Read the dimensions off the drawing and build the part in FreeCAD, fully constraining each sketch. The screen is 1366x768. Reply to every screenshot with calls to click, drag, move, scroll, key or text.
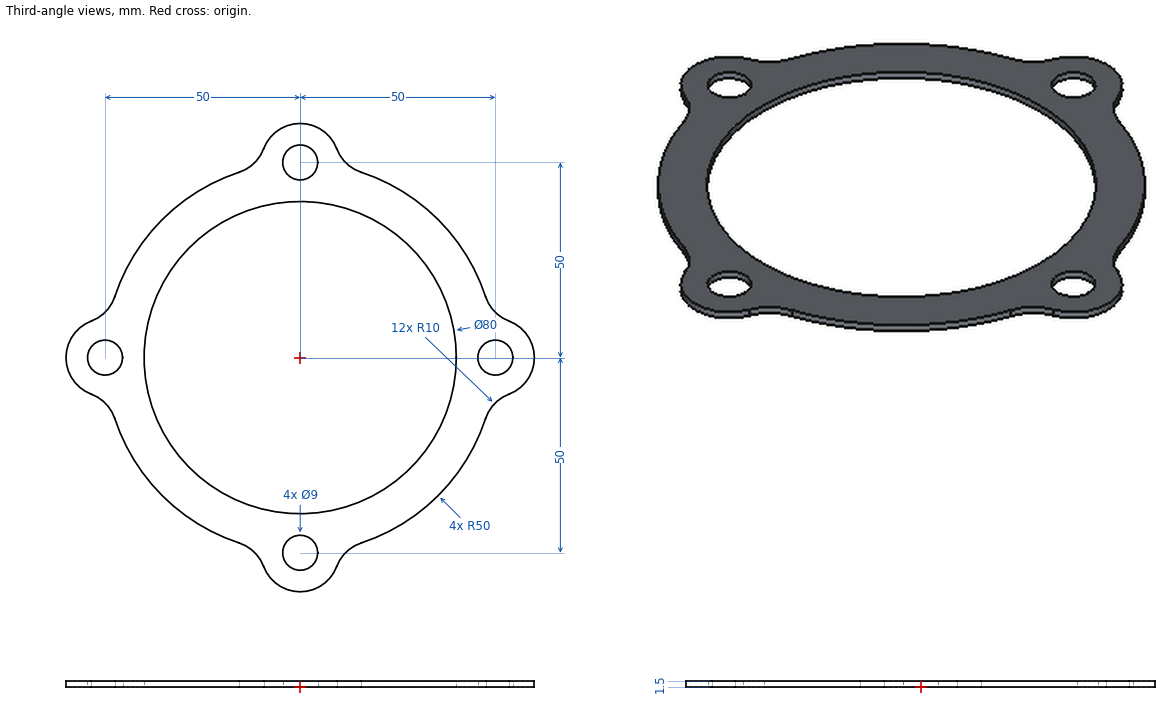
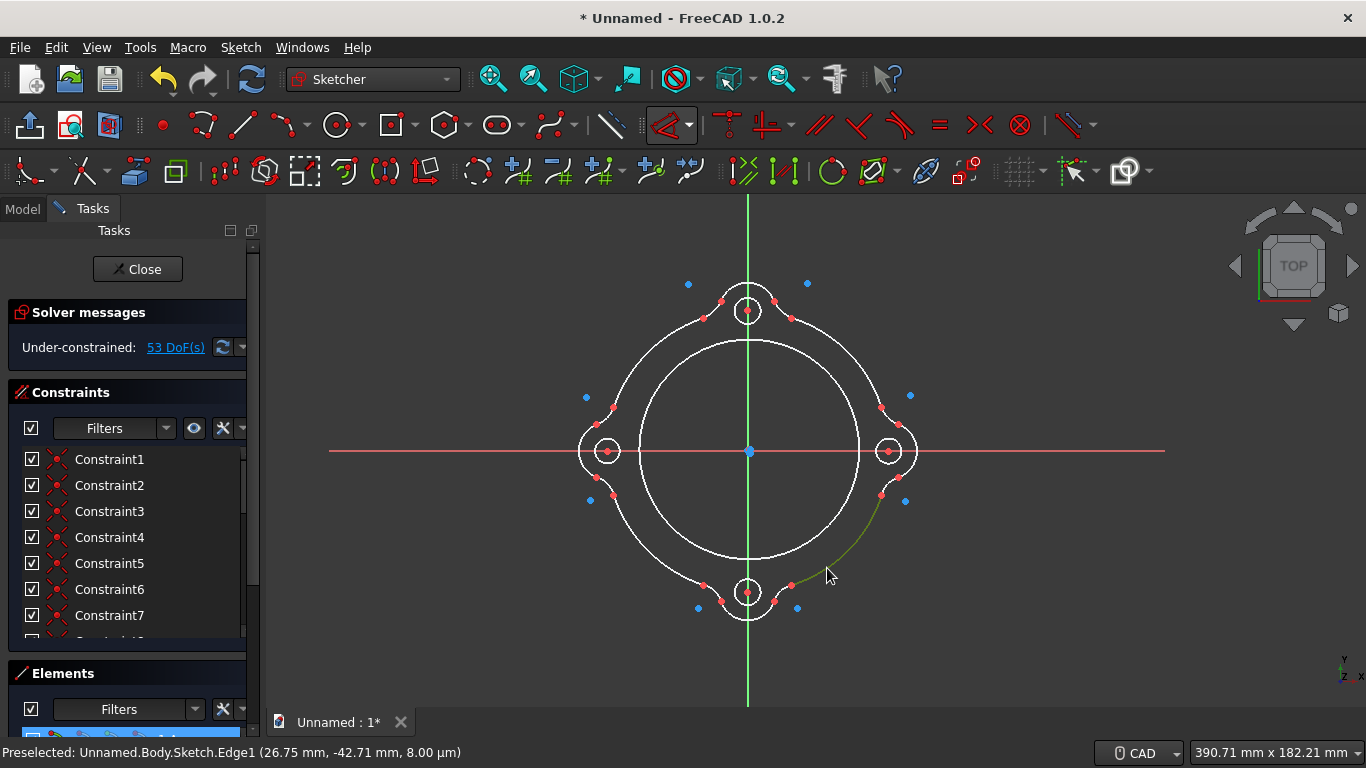
click(888, 484)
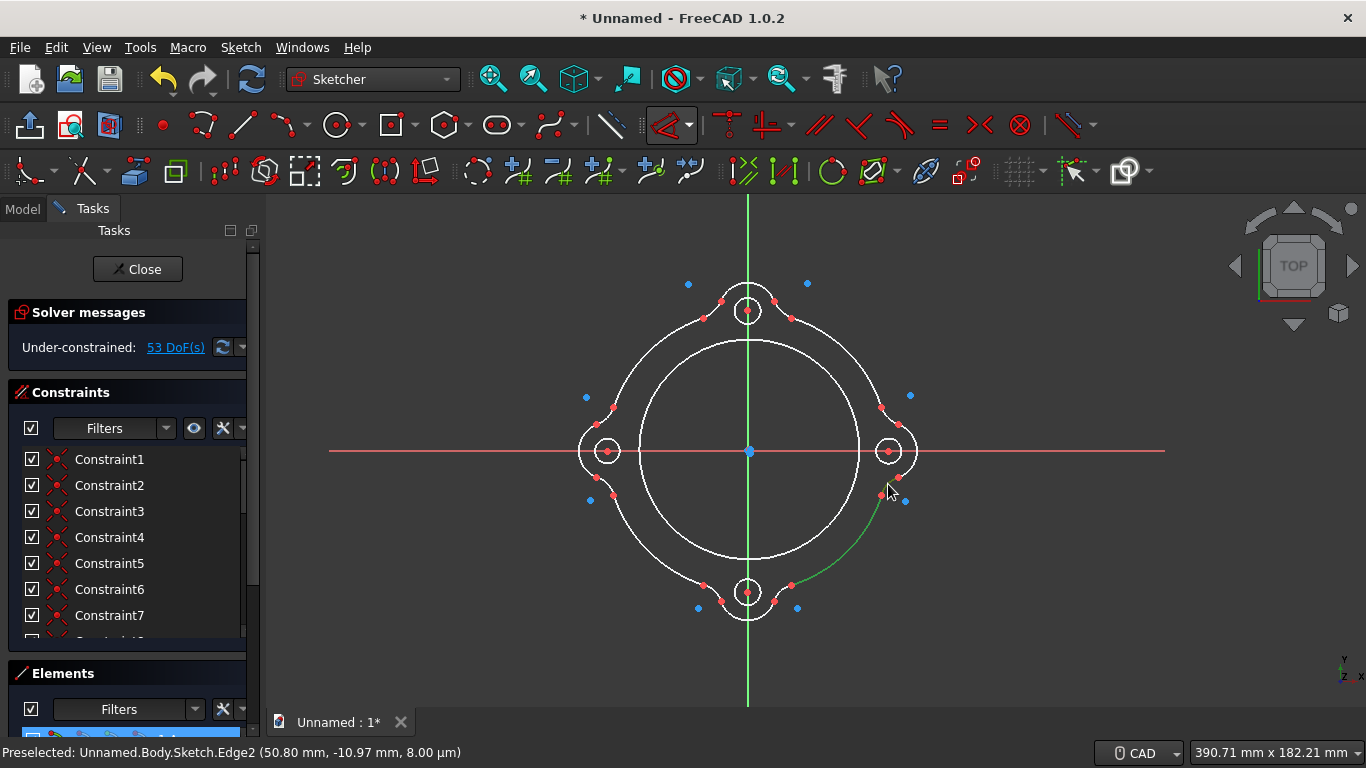
click(900, 126)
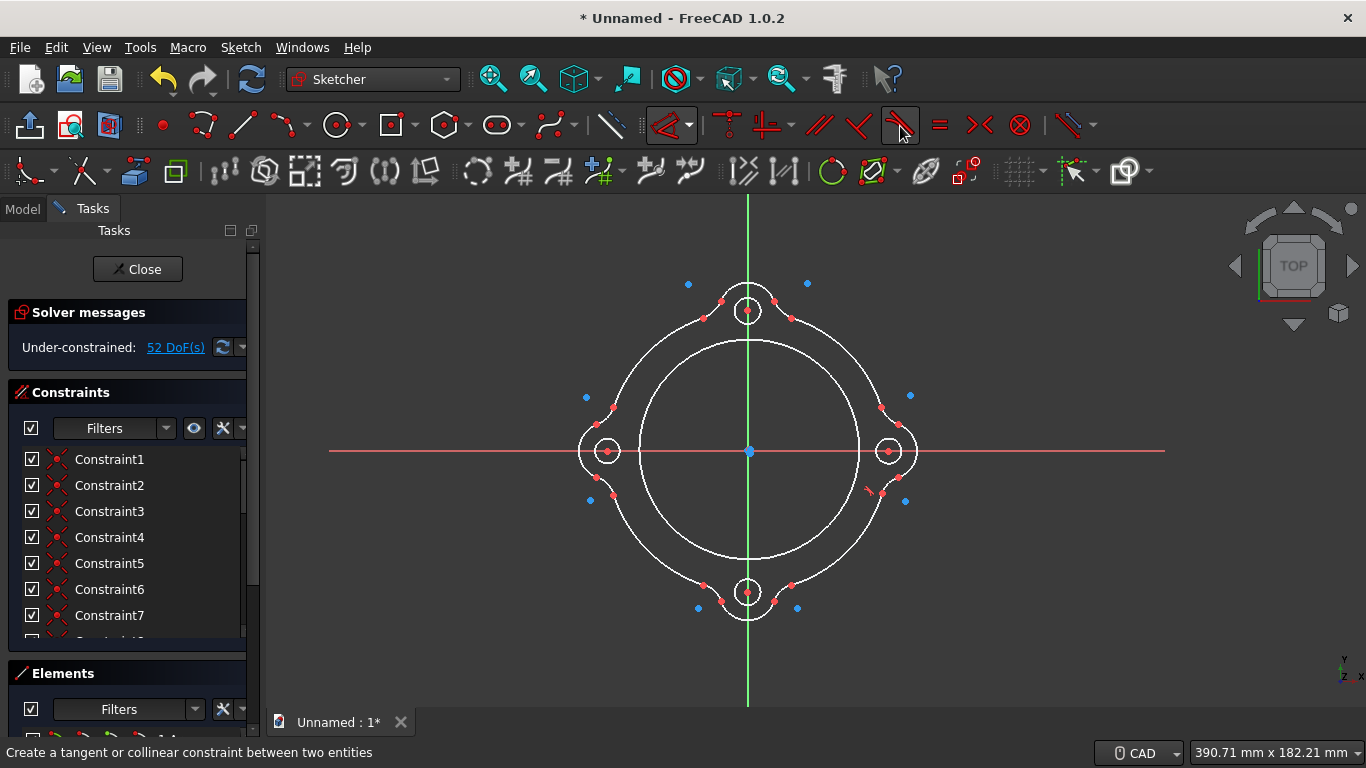
click(828, 568)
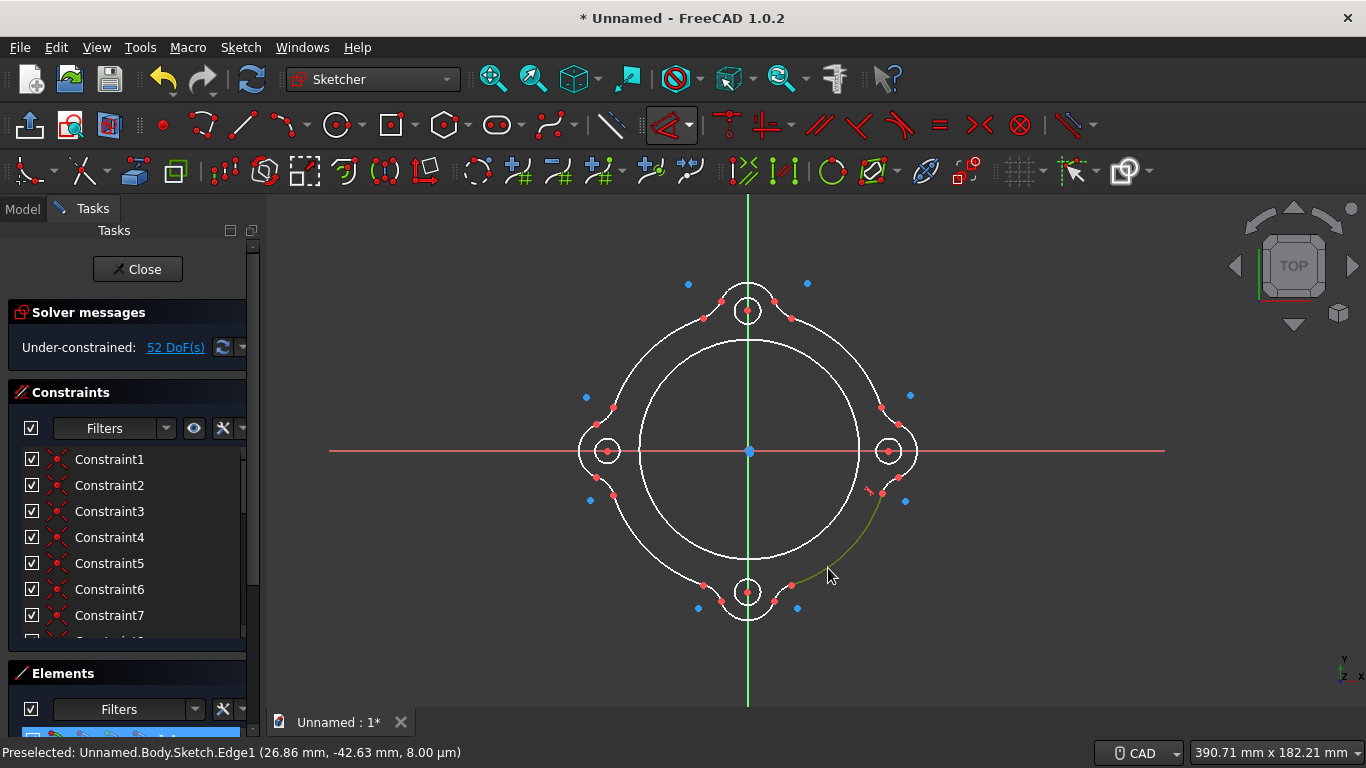
click(781, 591)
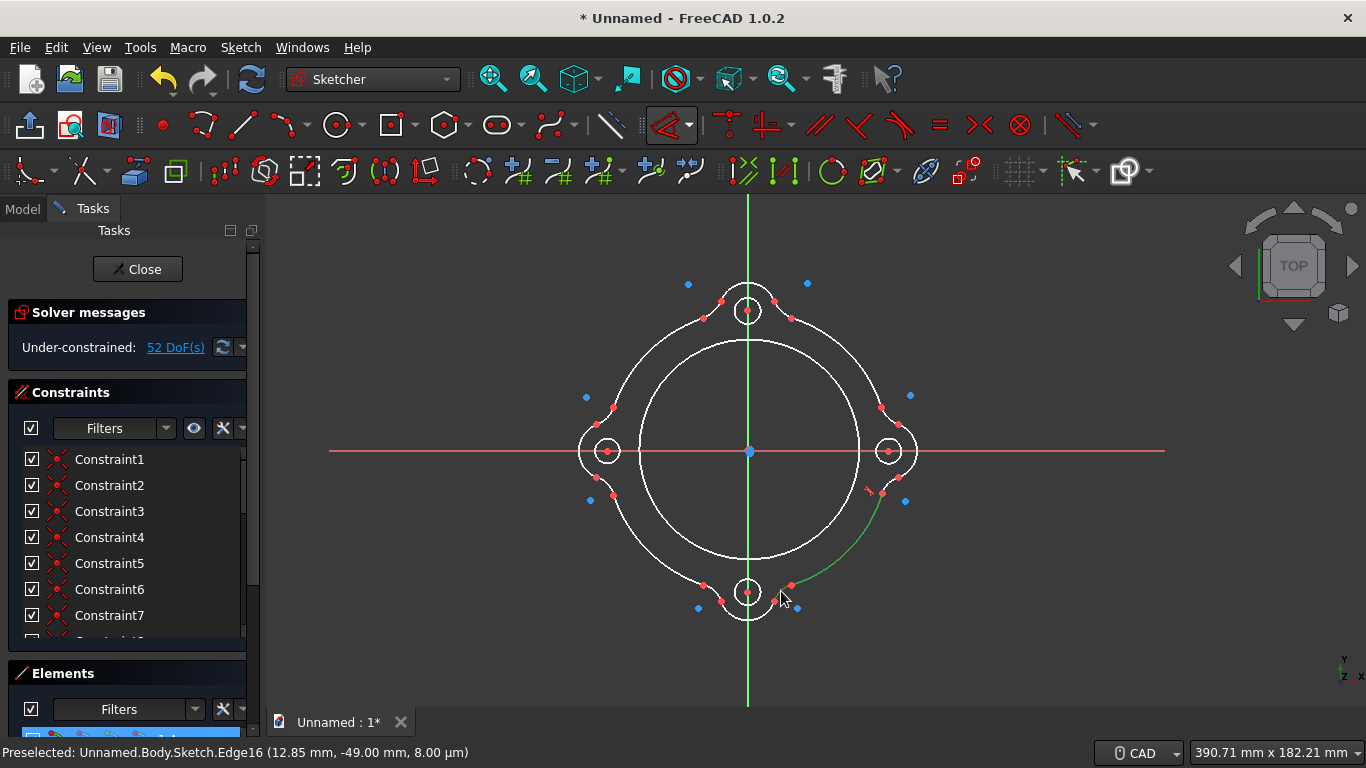
click(900, 126)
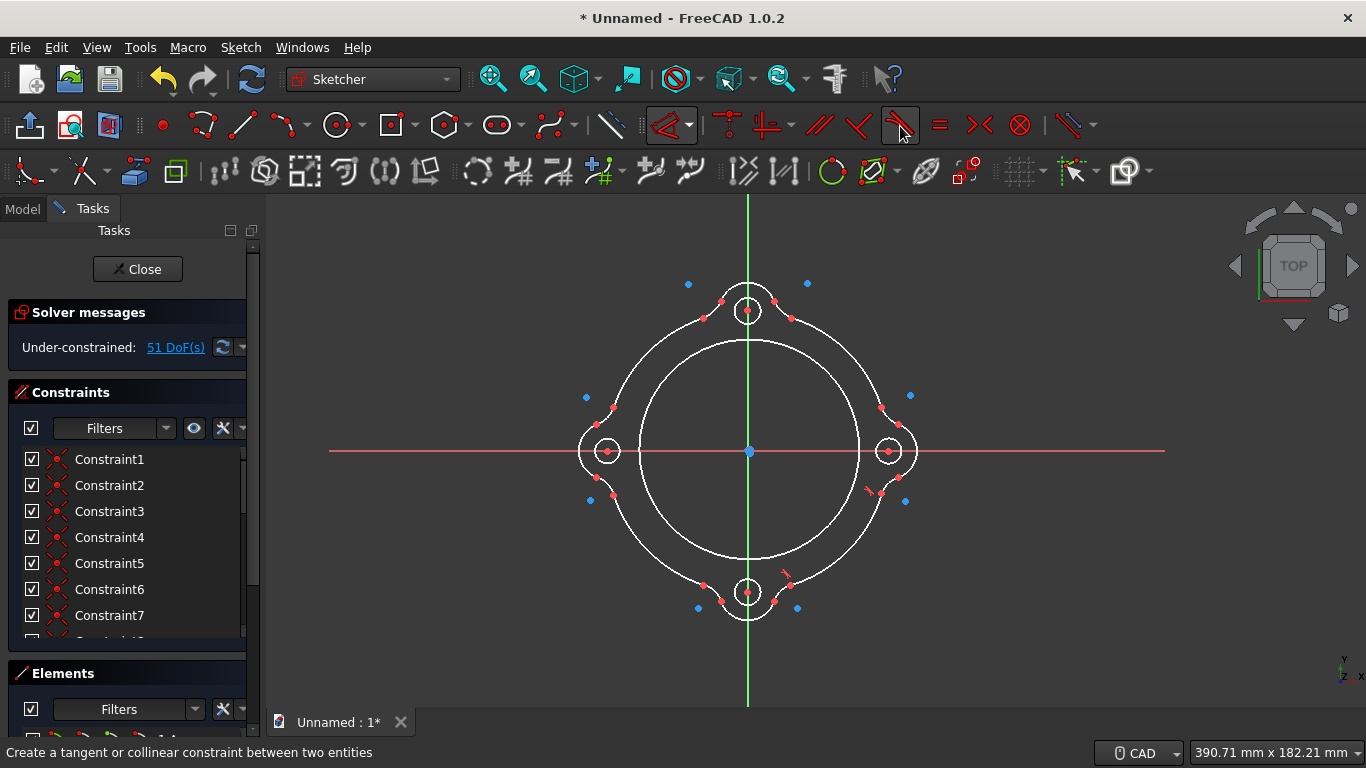
click(888, 484)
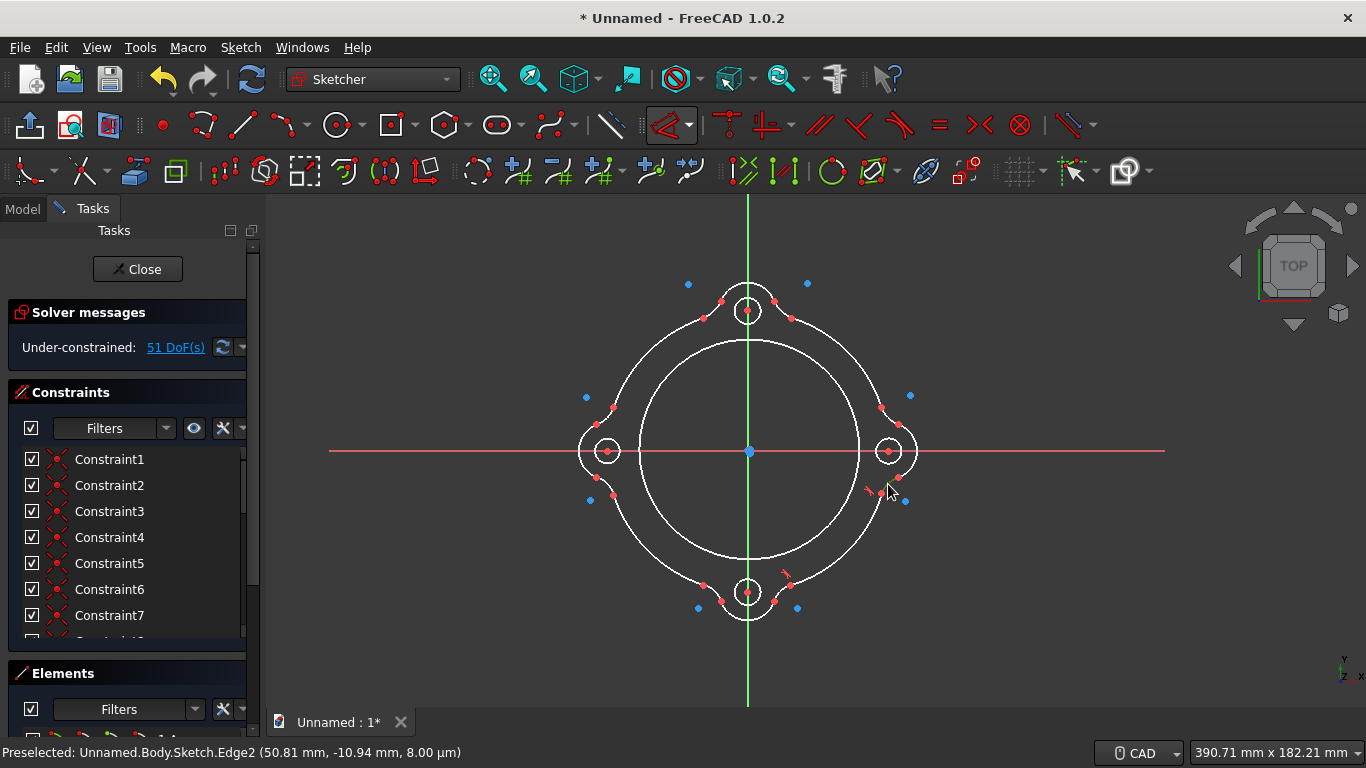
click(914, 464)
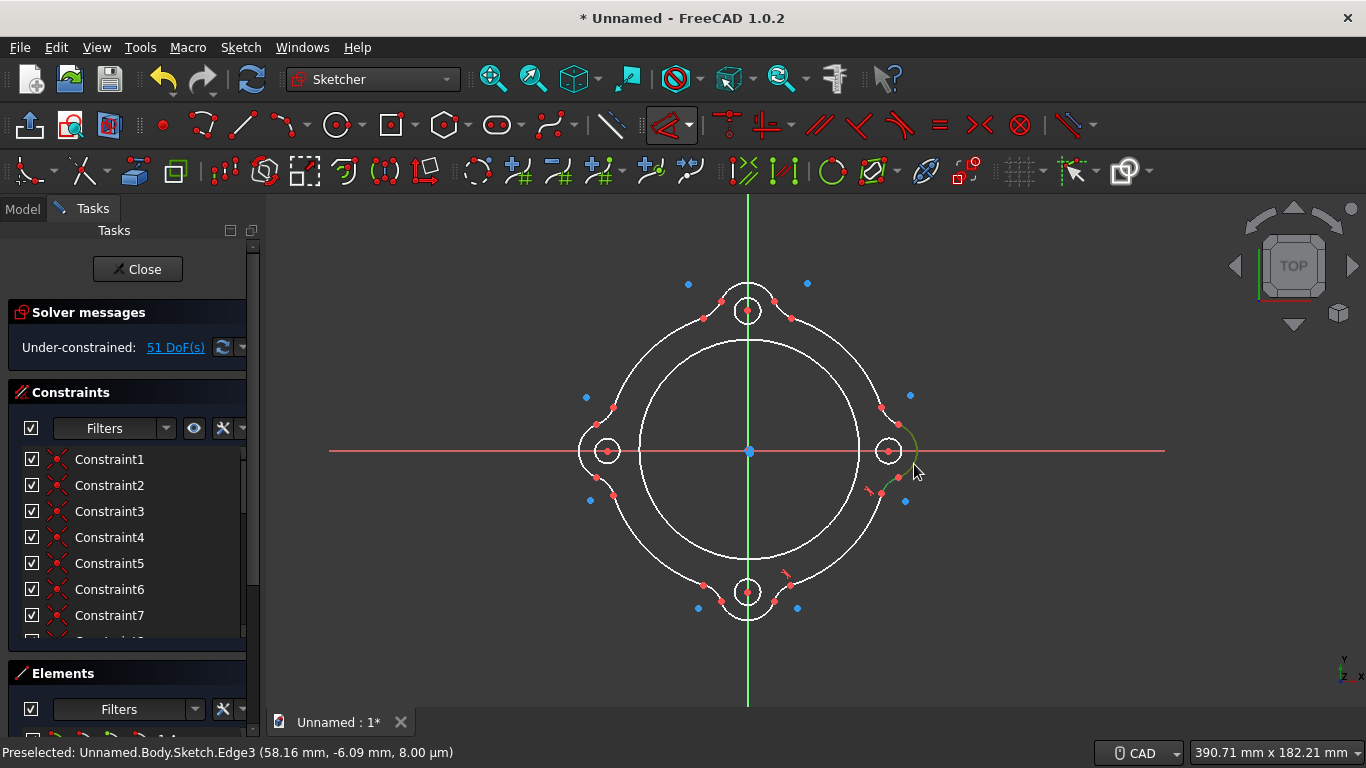
click(900, 126)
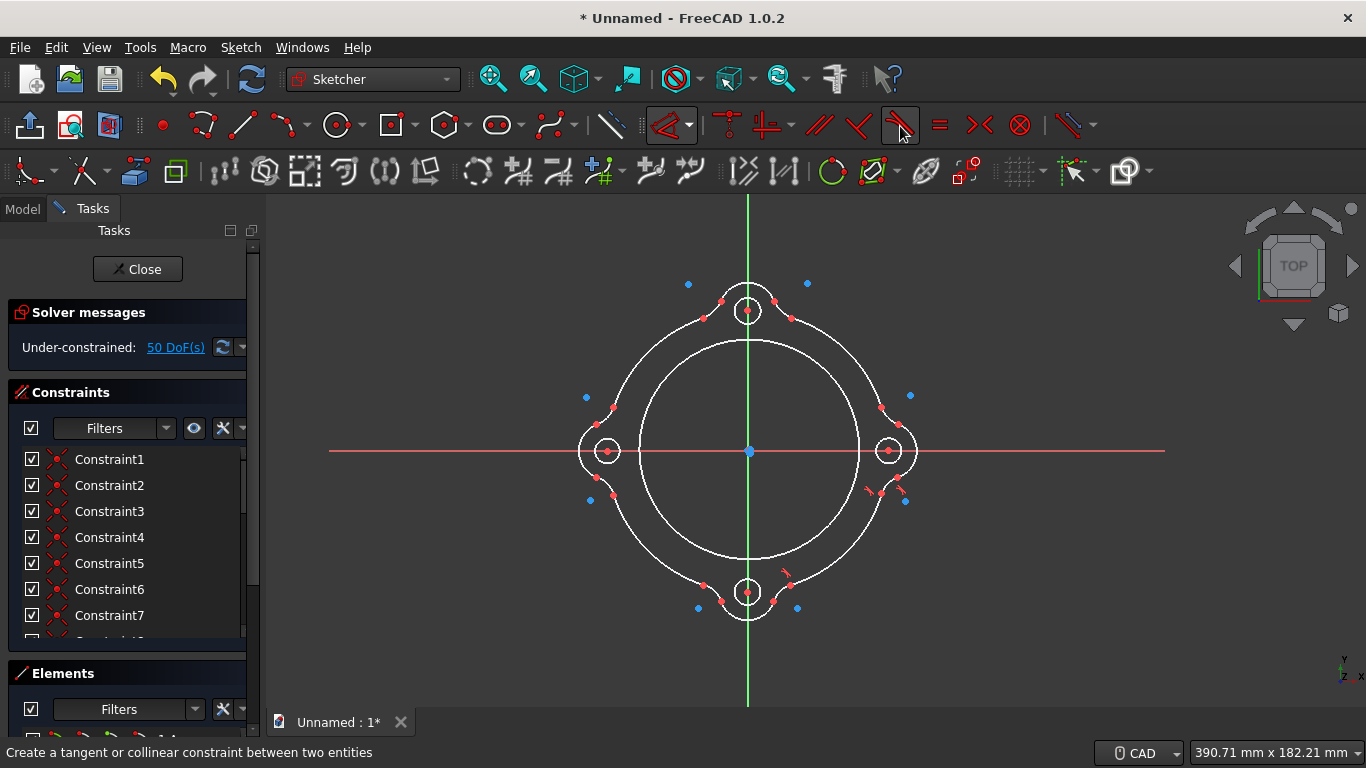
click(913, 465)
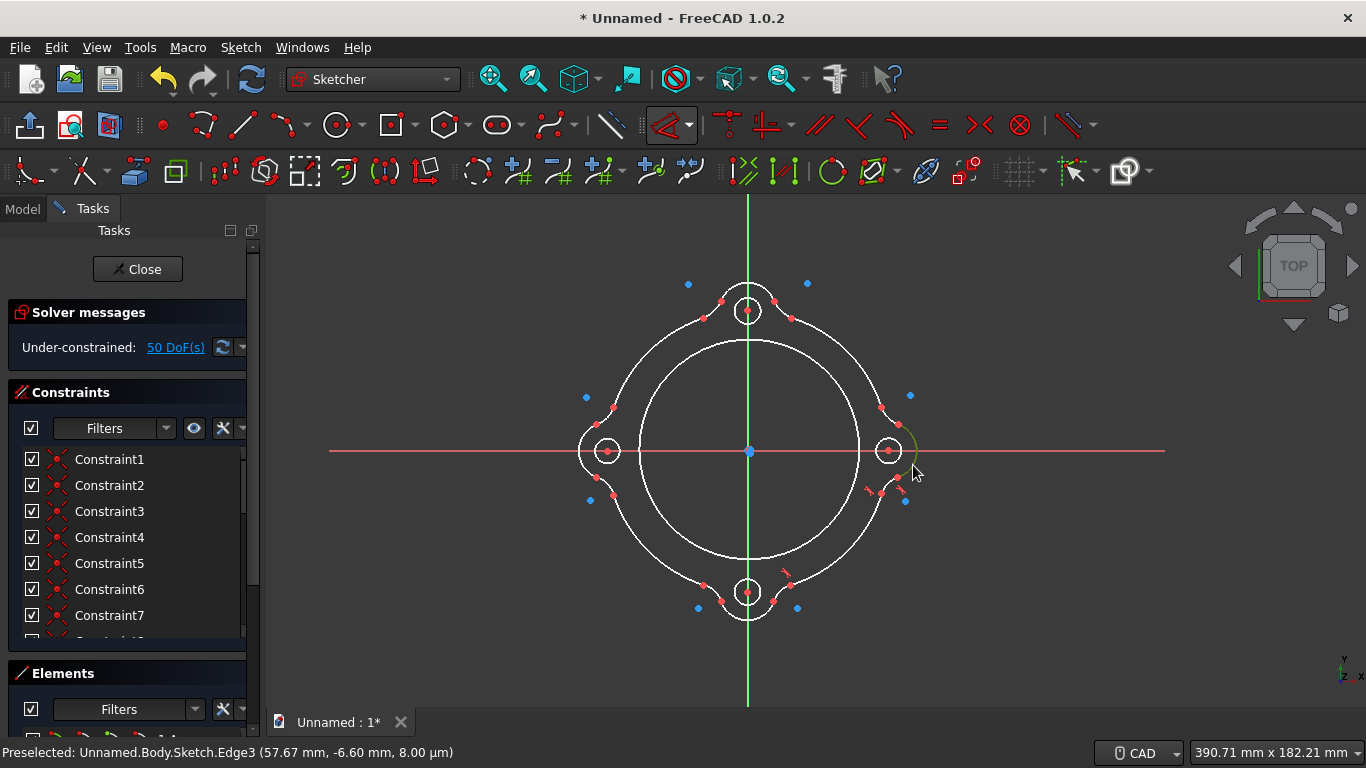
click(888, 418)